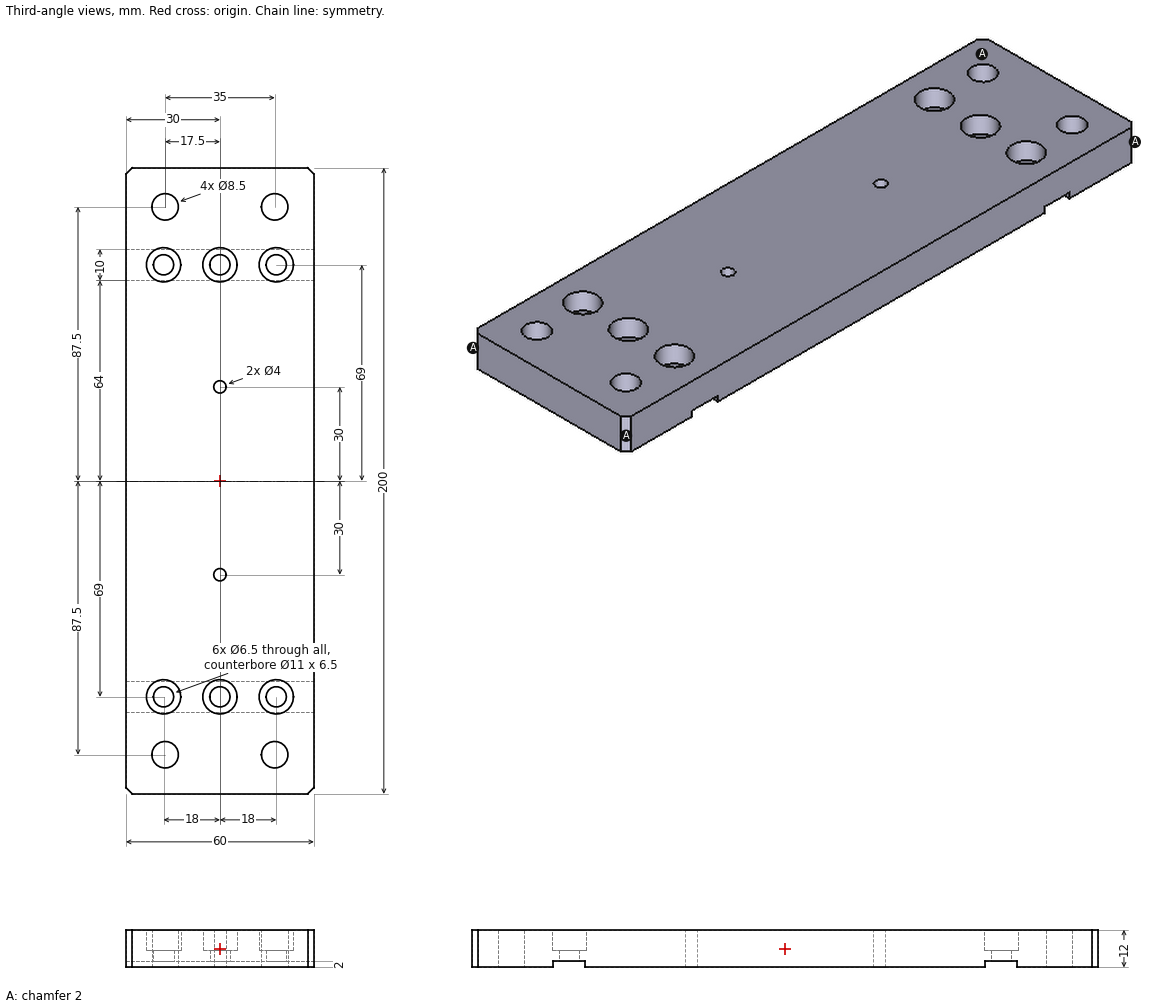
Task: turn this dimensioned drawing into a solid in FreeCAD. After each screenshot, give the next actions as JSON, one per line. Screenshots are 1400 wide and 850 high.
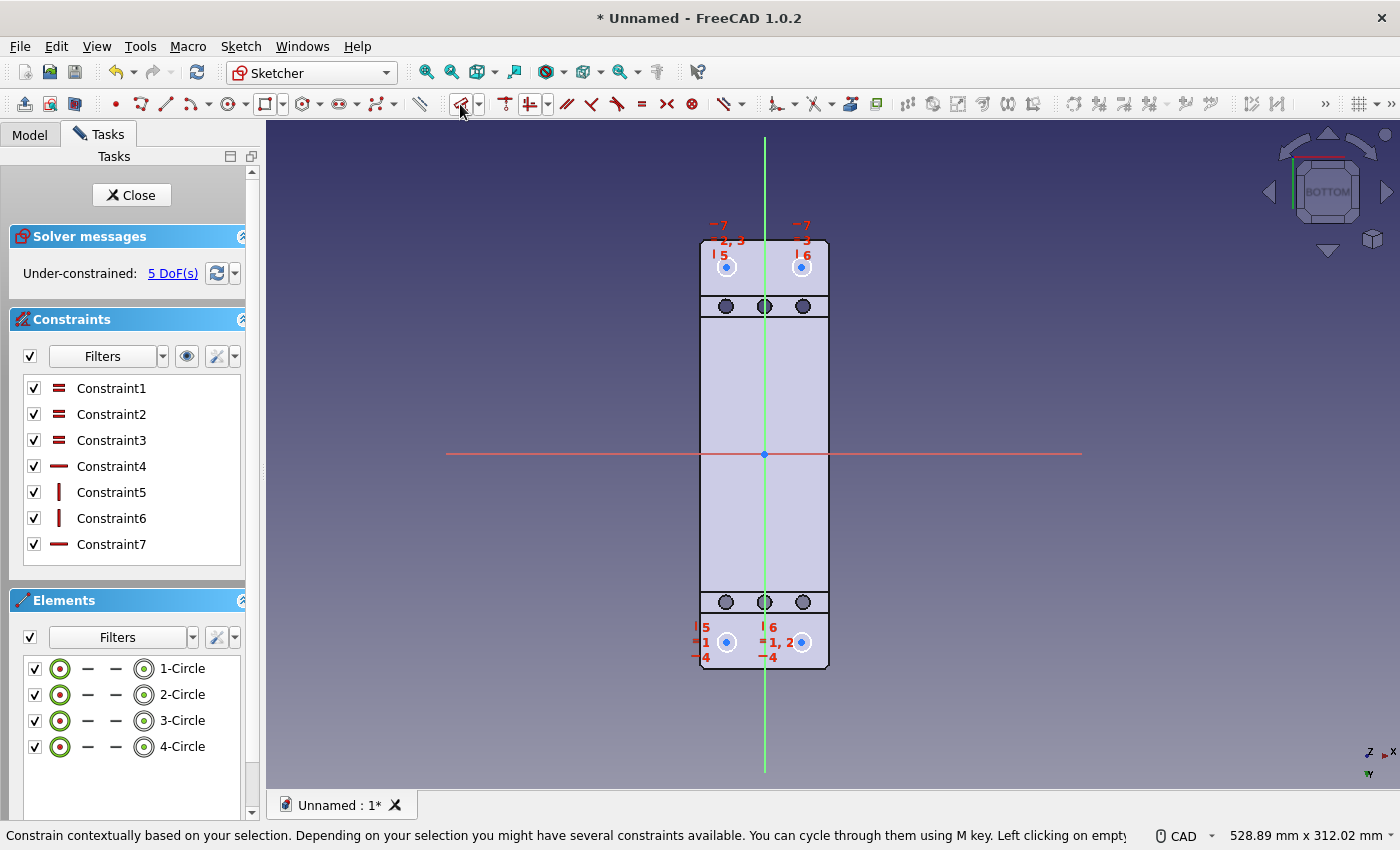
{"action": "scroll", "coordinate": [733, 636], "scroll_direction": "up", "scroll_amount": 4}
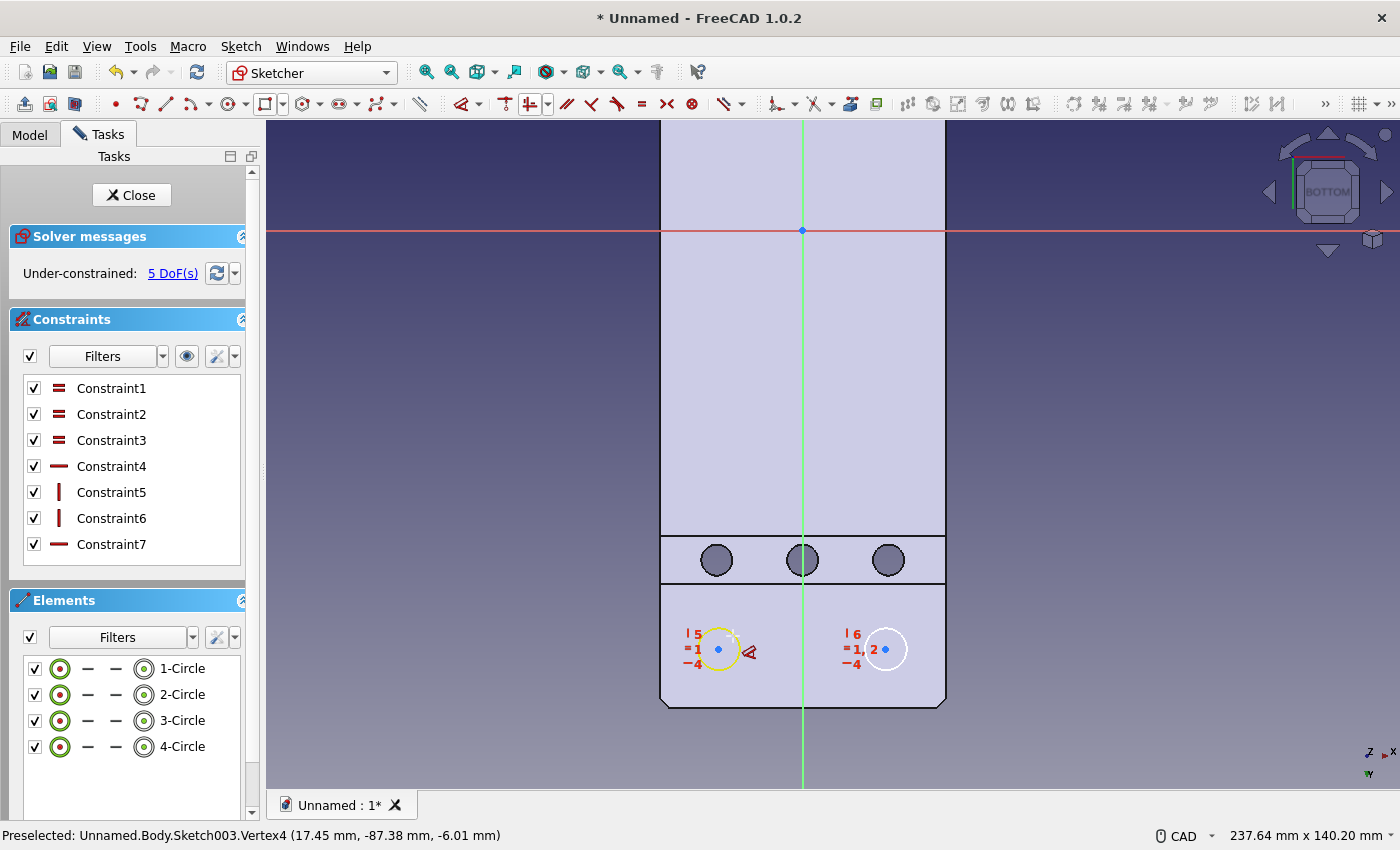
{"action": "left_click", "coordinate": [734, 634]}
{"action": "left_click", "coordinate": [757, 611]}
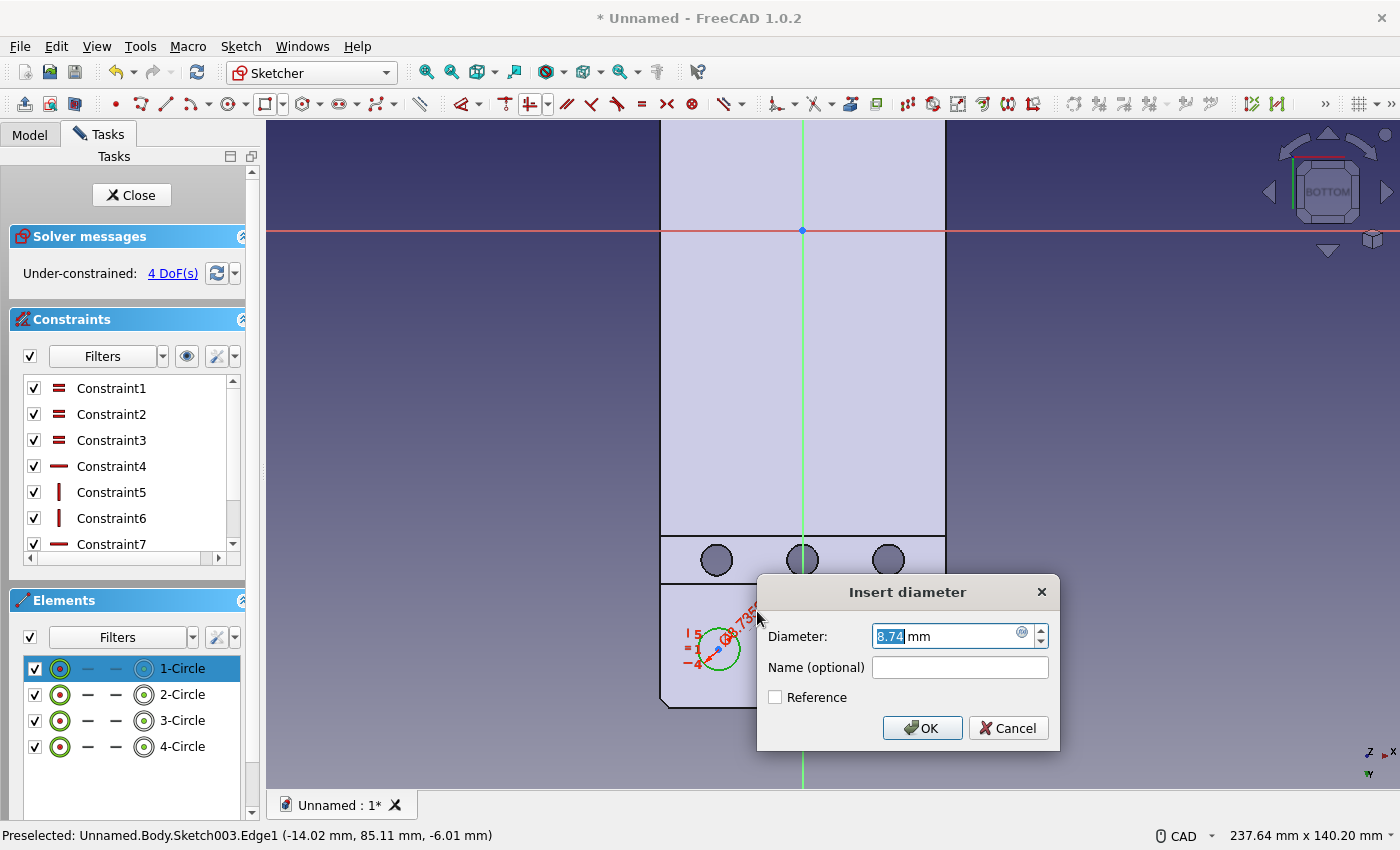
{"action": "type", "text": "8.5"}
{"action": "key", "text": "Return"}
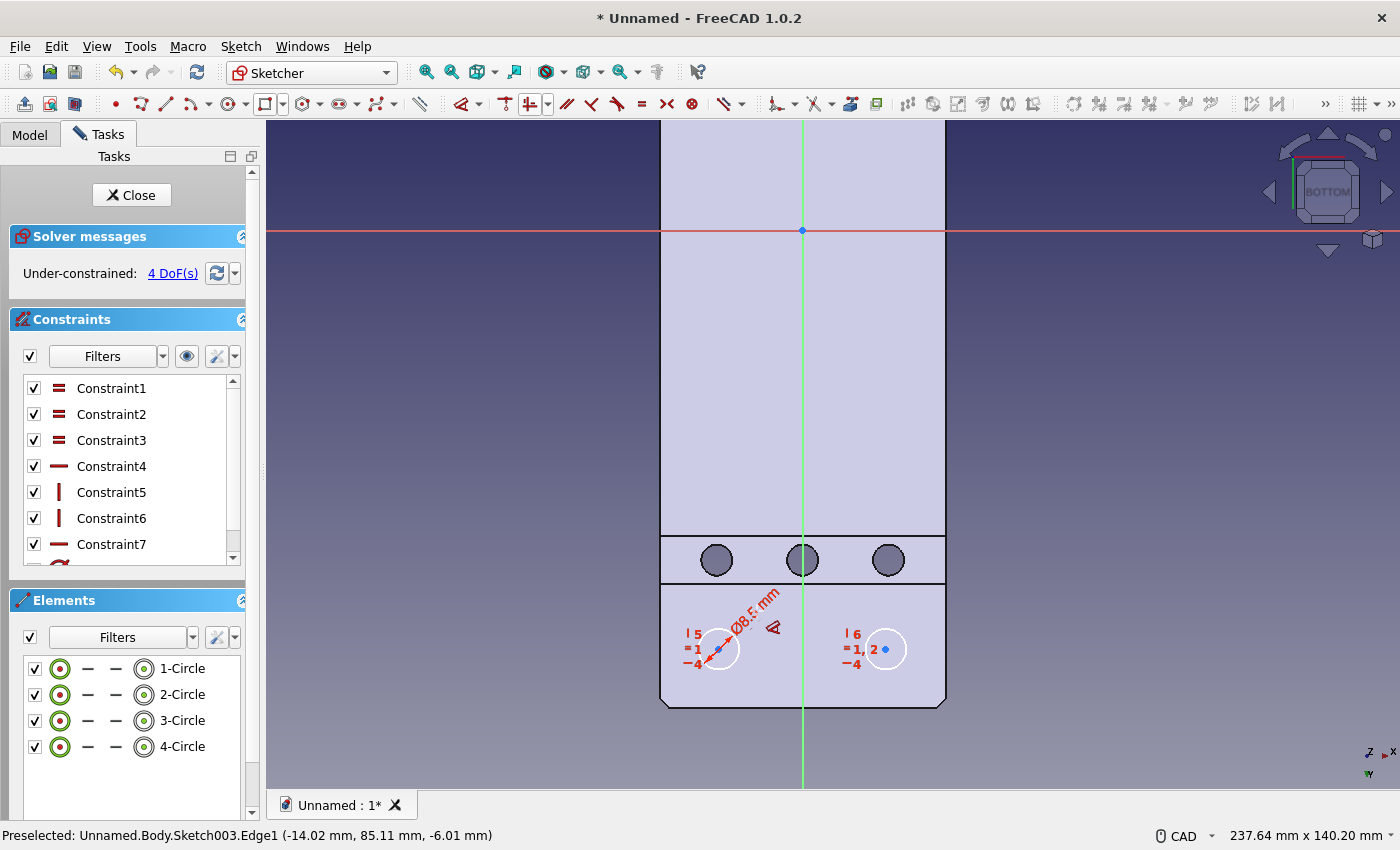
{"action": "left_click", "coordinate": [719, 649]}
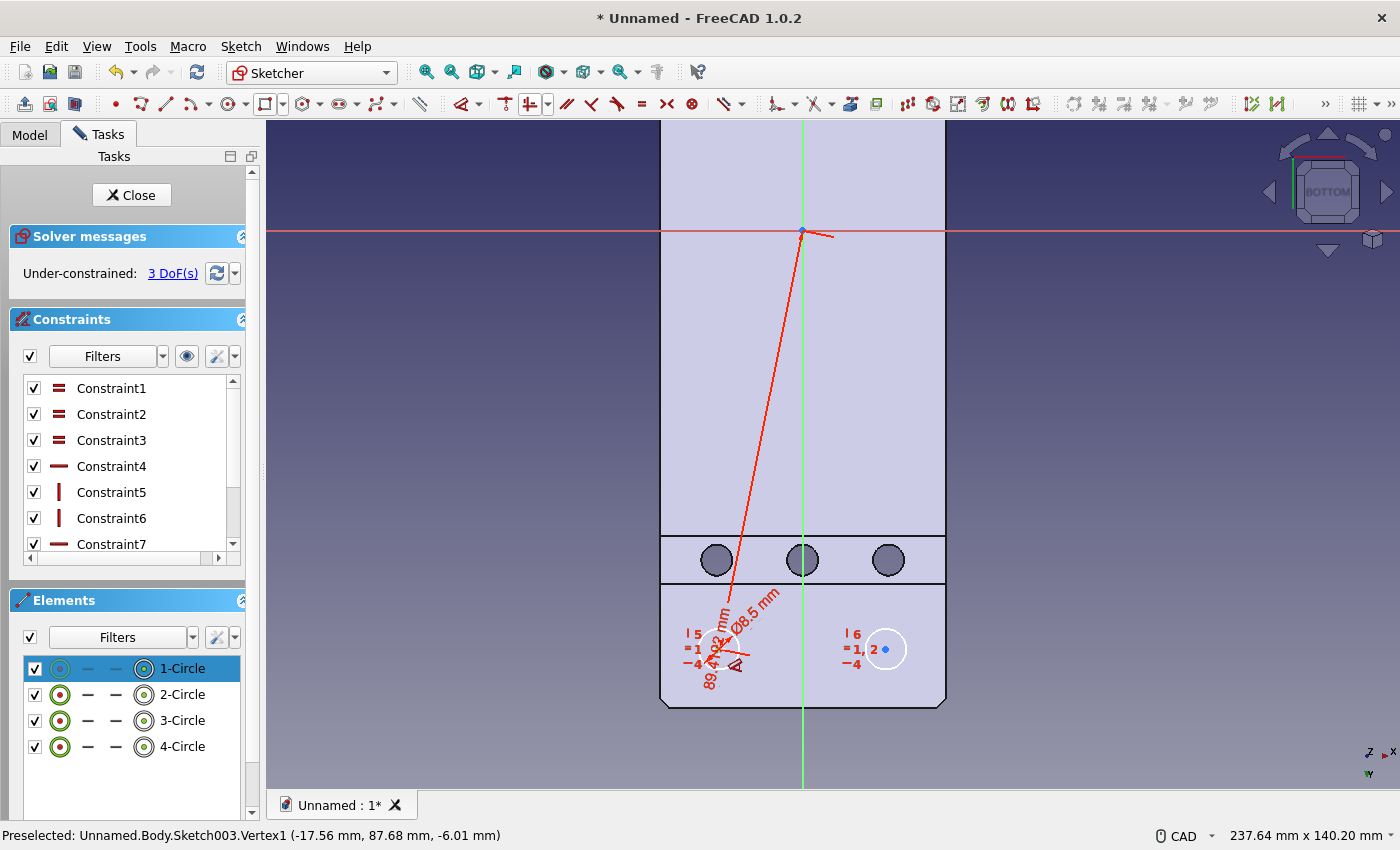
{"action": "left_click", "coordinate": [886, 649]}
{"action": "left_click", "coordinate": [764, 683]}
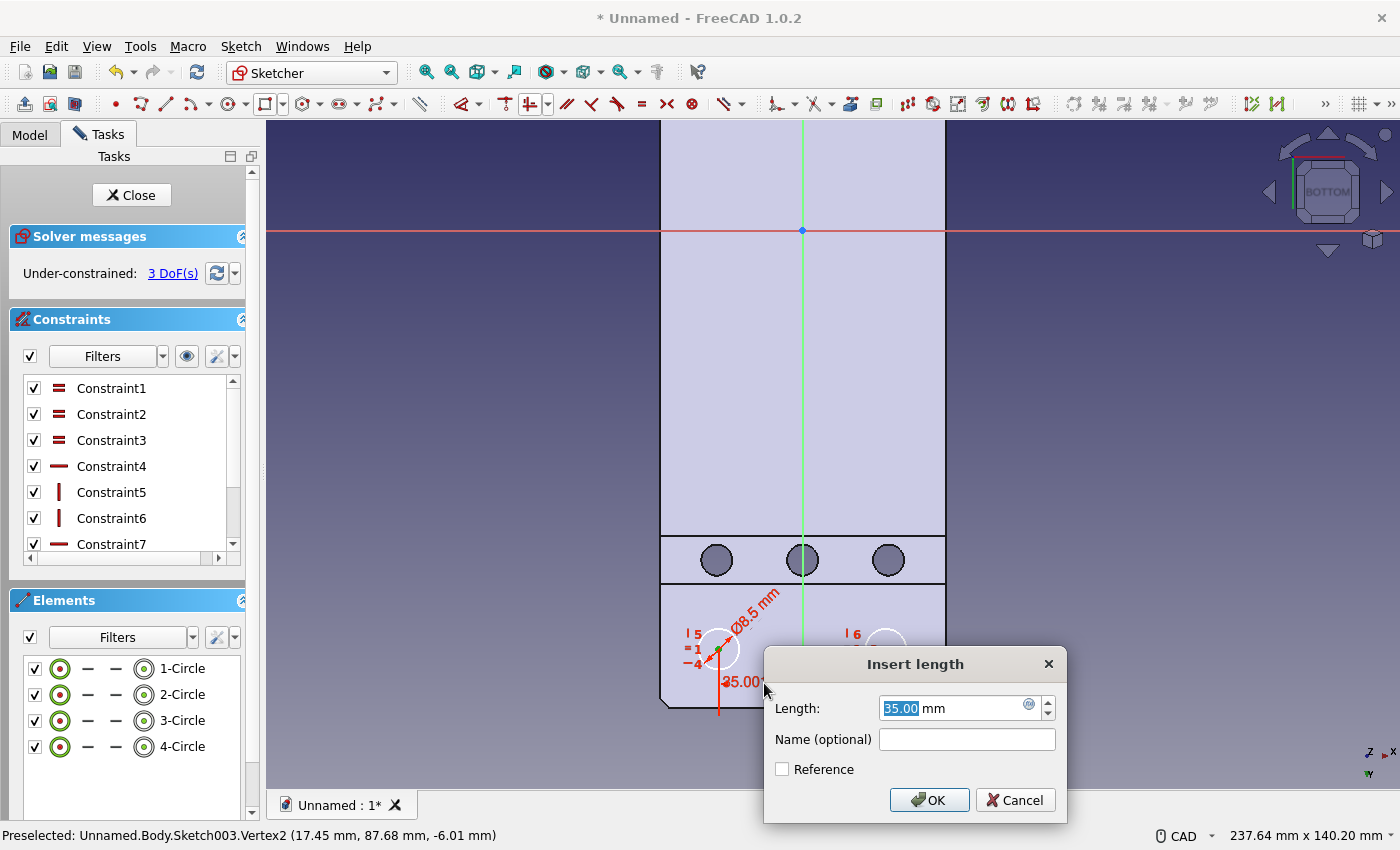
{"action": "type", "text": "35"}
{"action": "key", "text": "Return"}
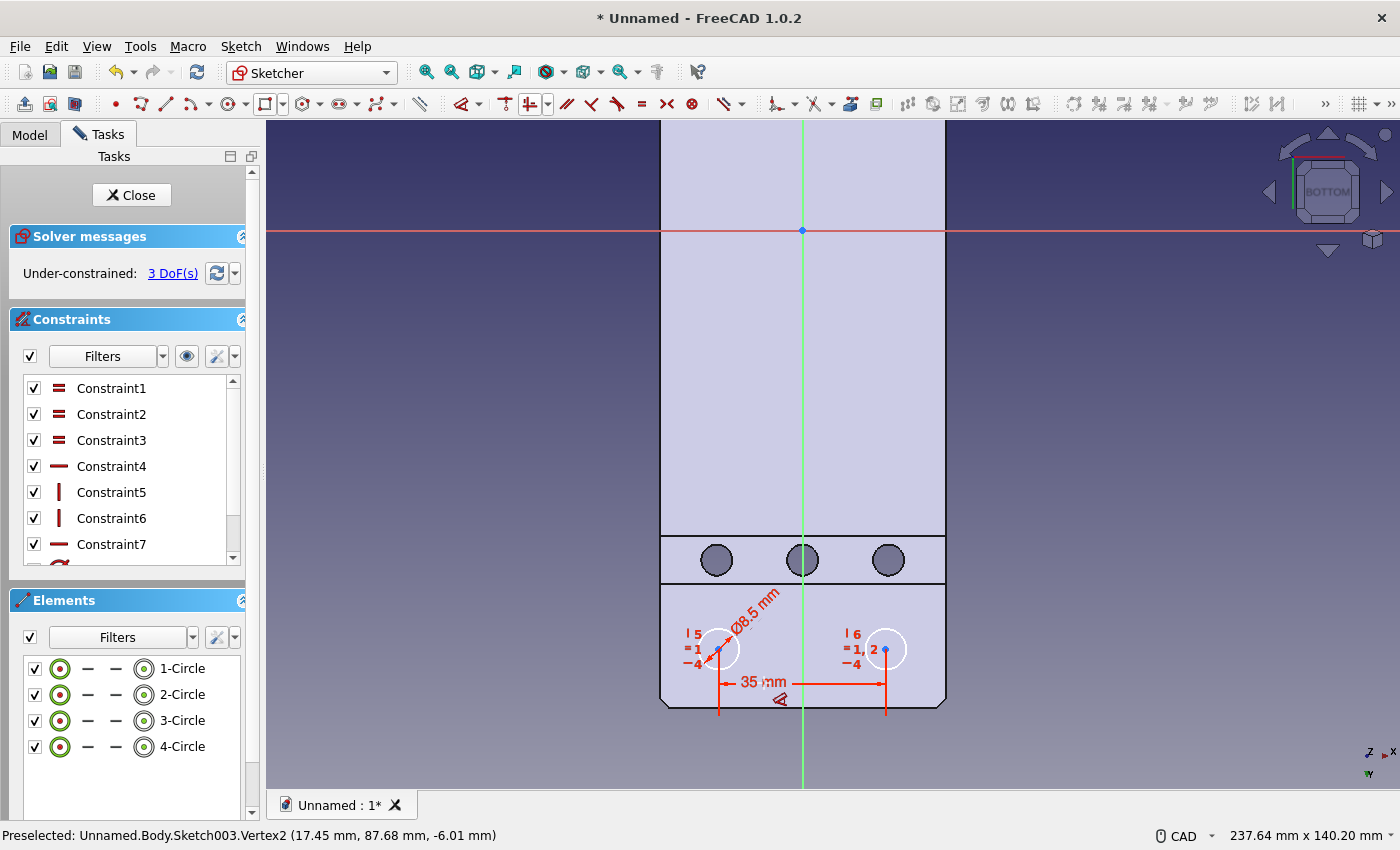
{"action": "left_click", "coordinate": [719, 649]}
{"action": "left_click", "coordinate": [761, 197]}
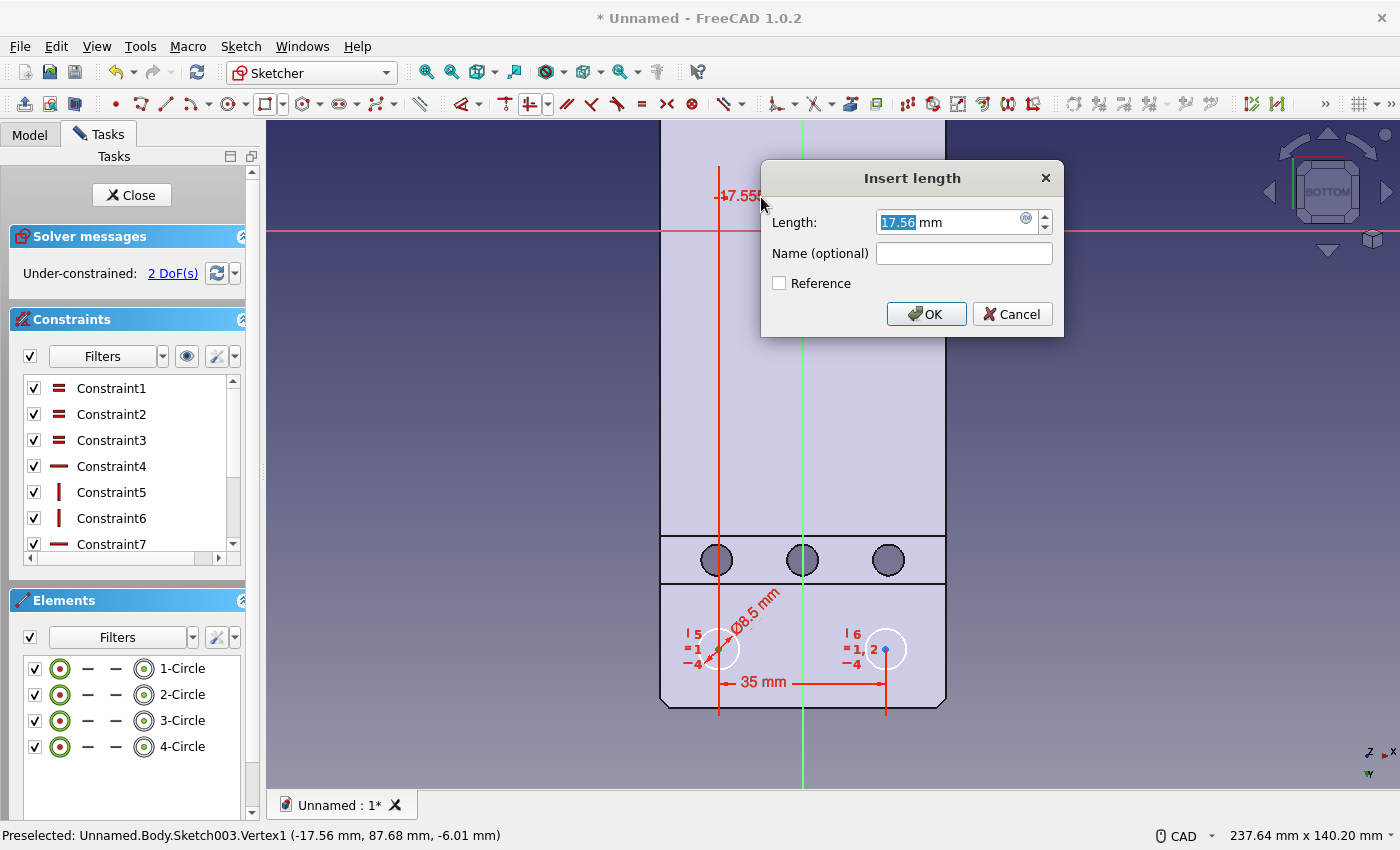
{"action": "type", "text": "17.5"}
{"action": "key", "text": "Return"}